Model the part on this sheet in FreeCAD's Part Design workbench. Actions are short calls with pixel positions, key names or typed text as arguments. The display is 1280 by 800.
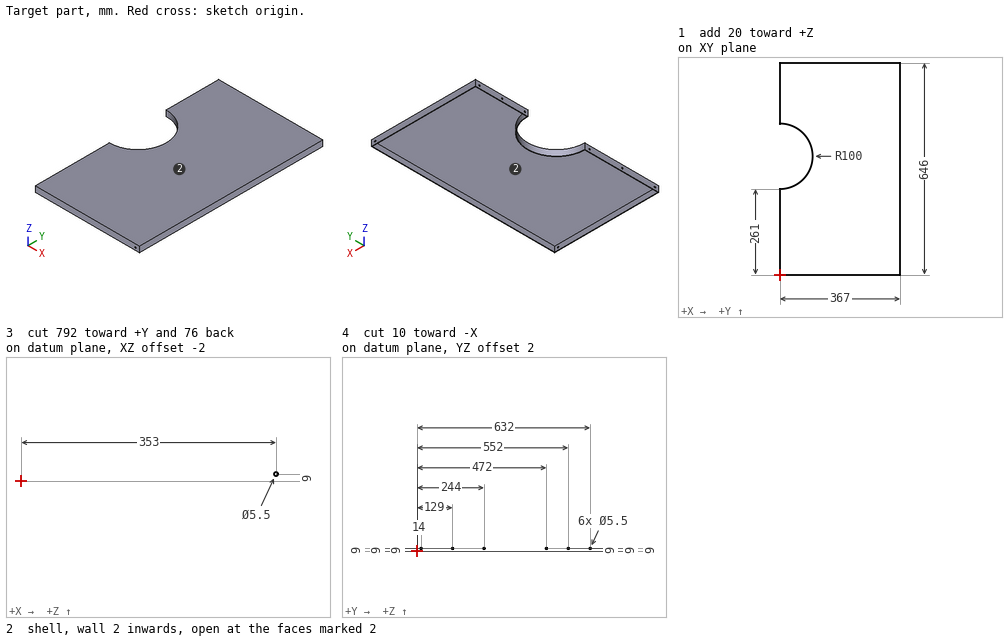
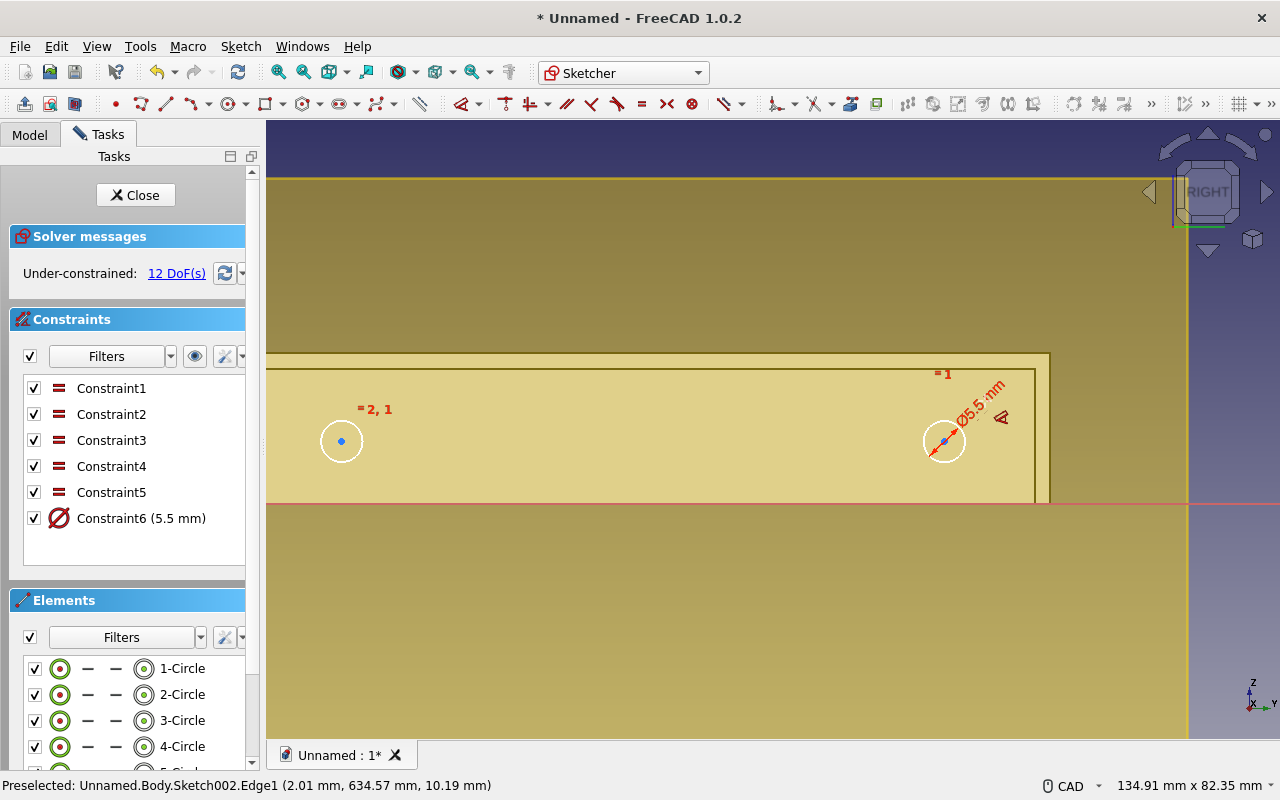
click(944, 442)
click(978, 473)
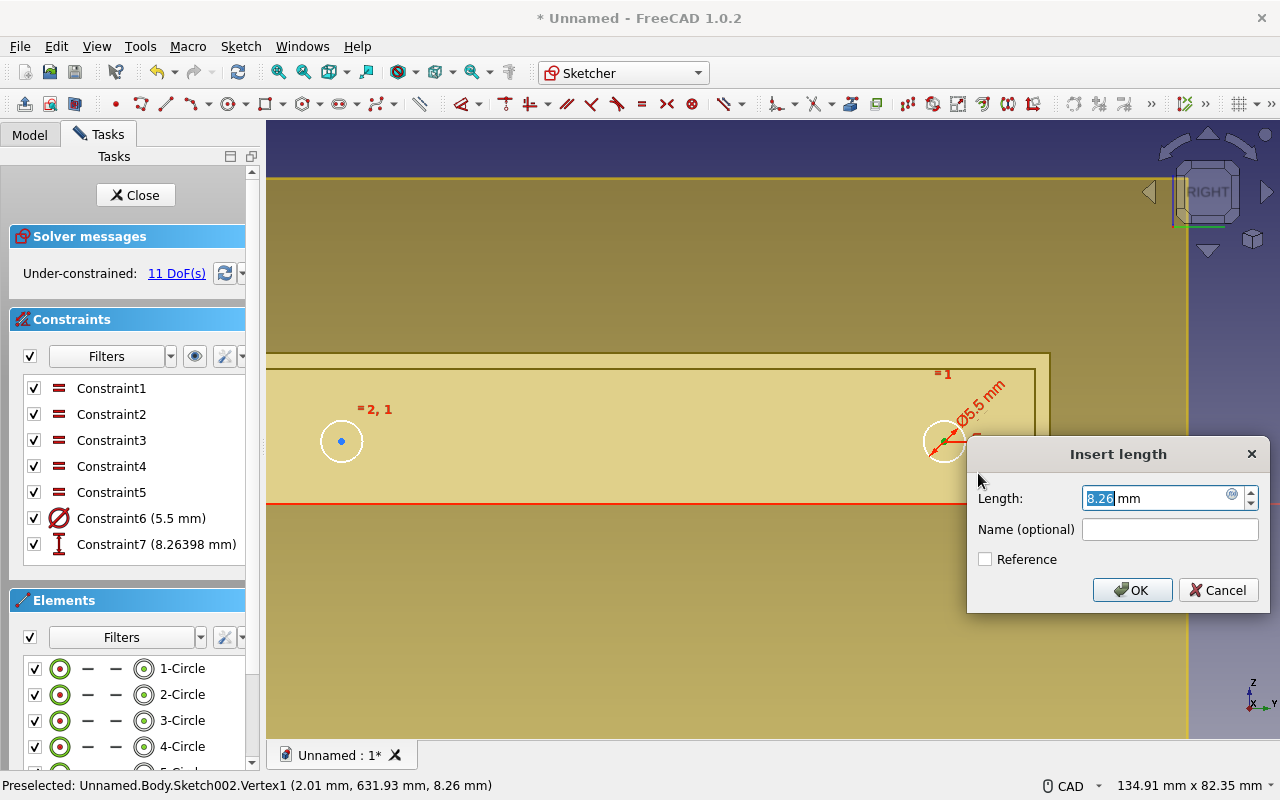
text(9)
key(Return)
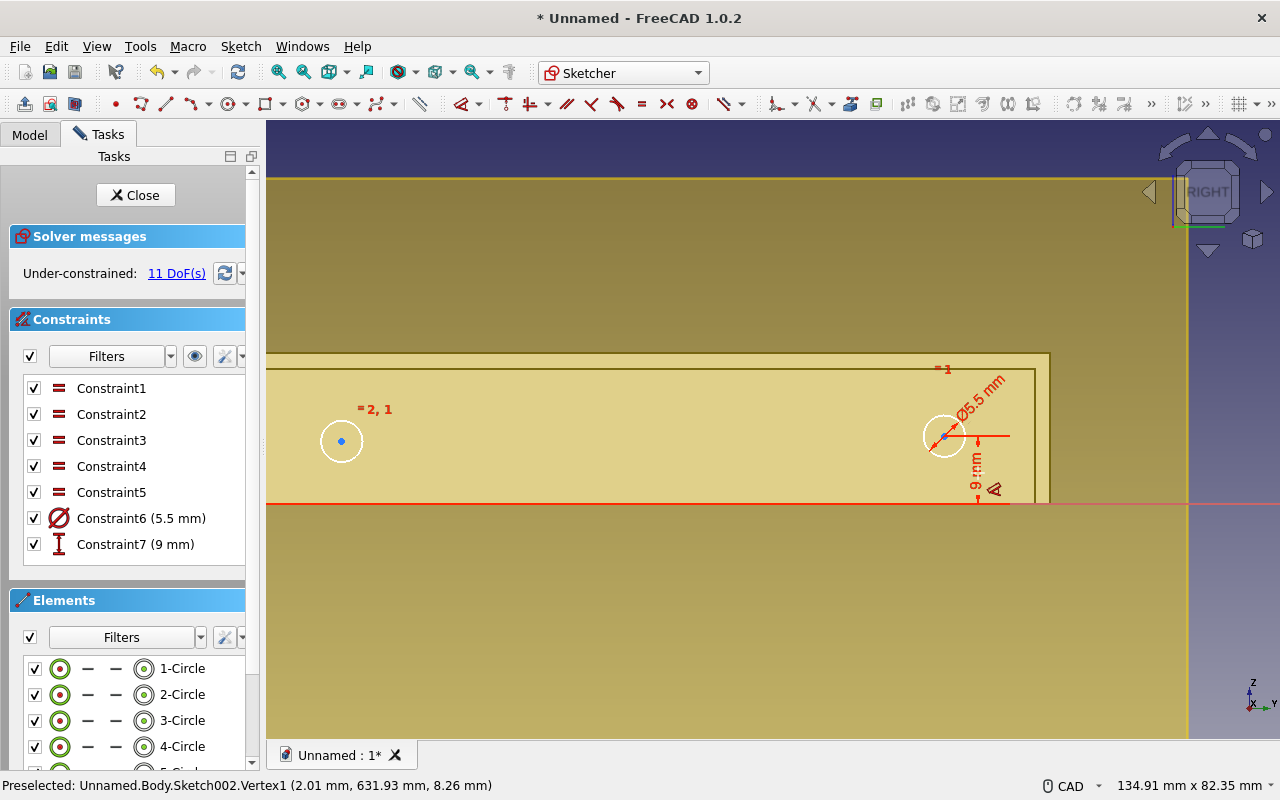
click(342, 441)
click(376, 473)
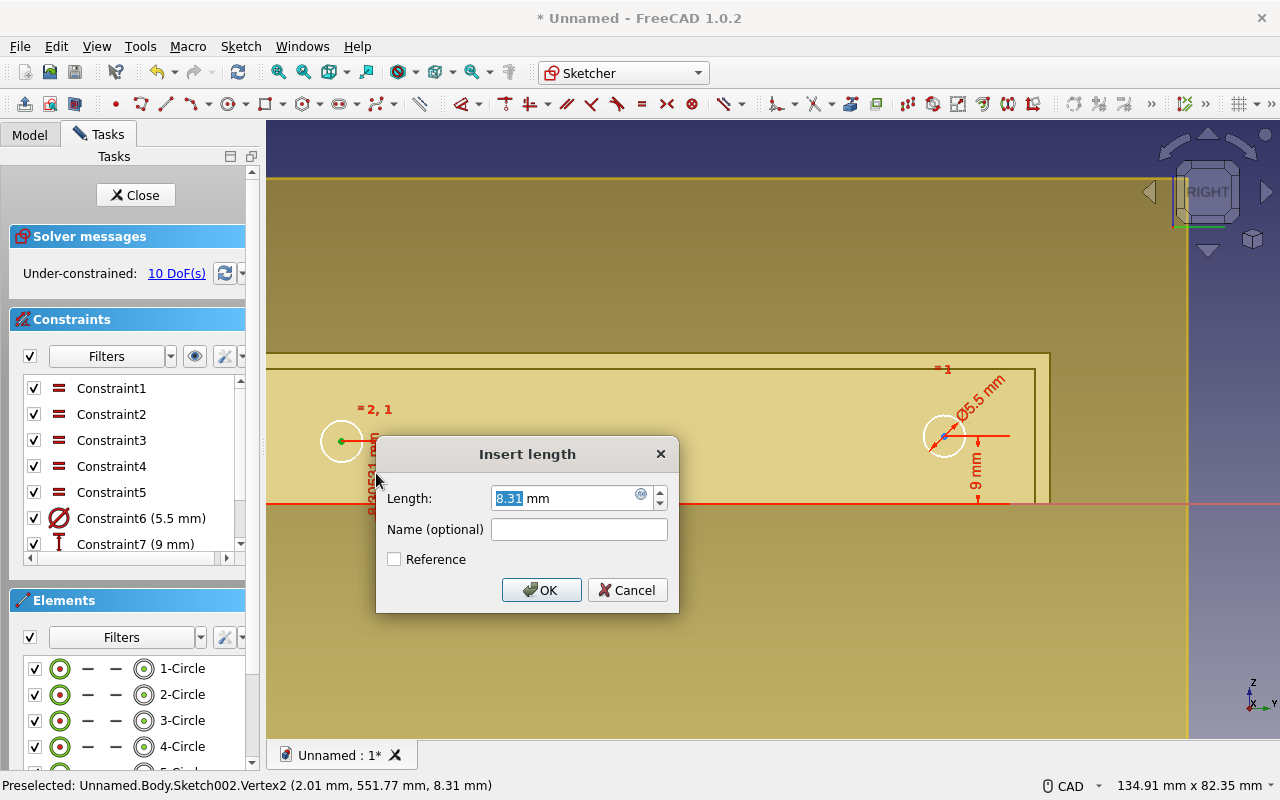
text(9)
key(Return)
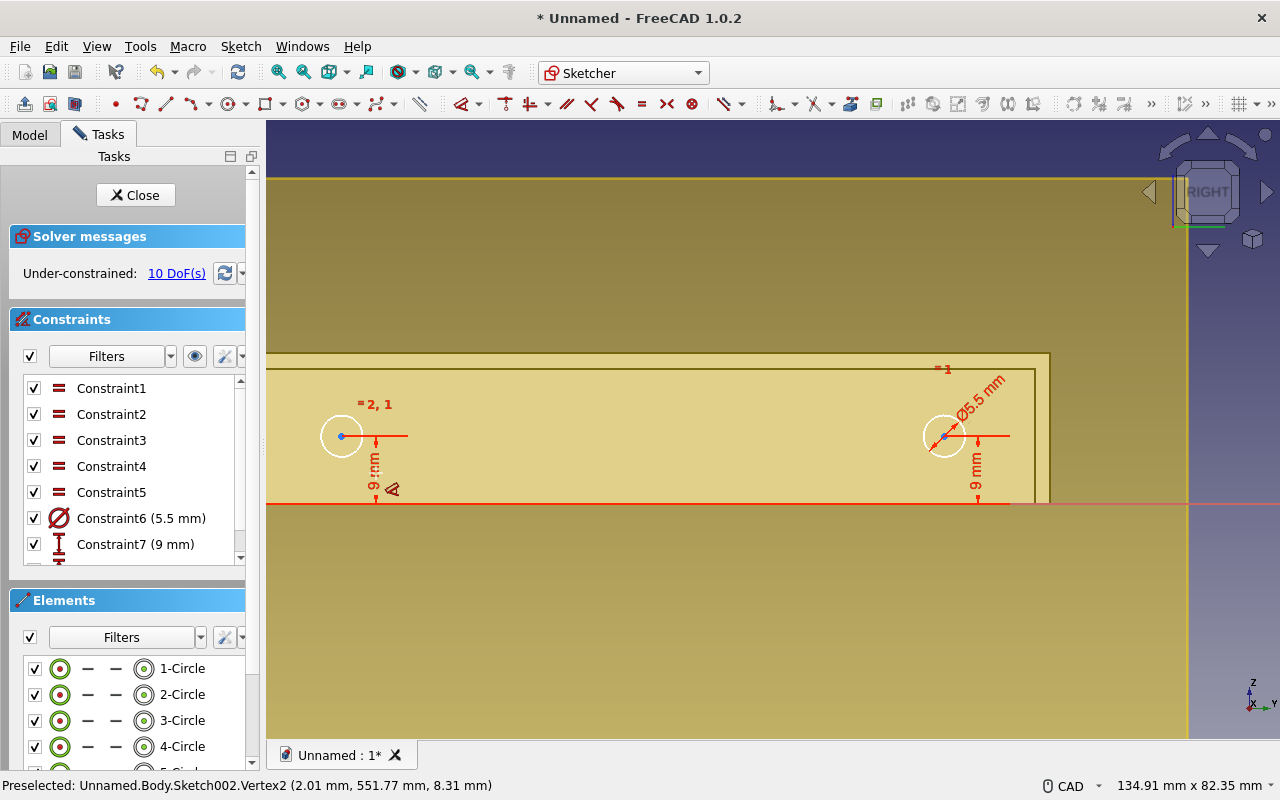
scroll(969, 426, down, 11)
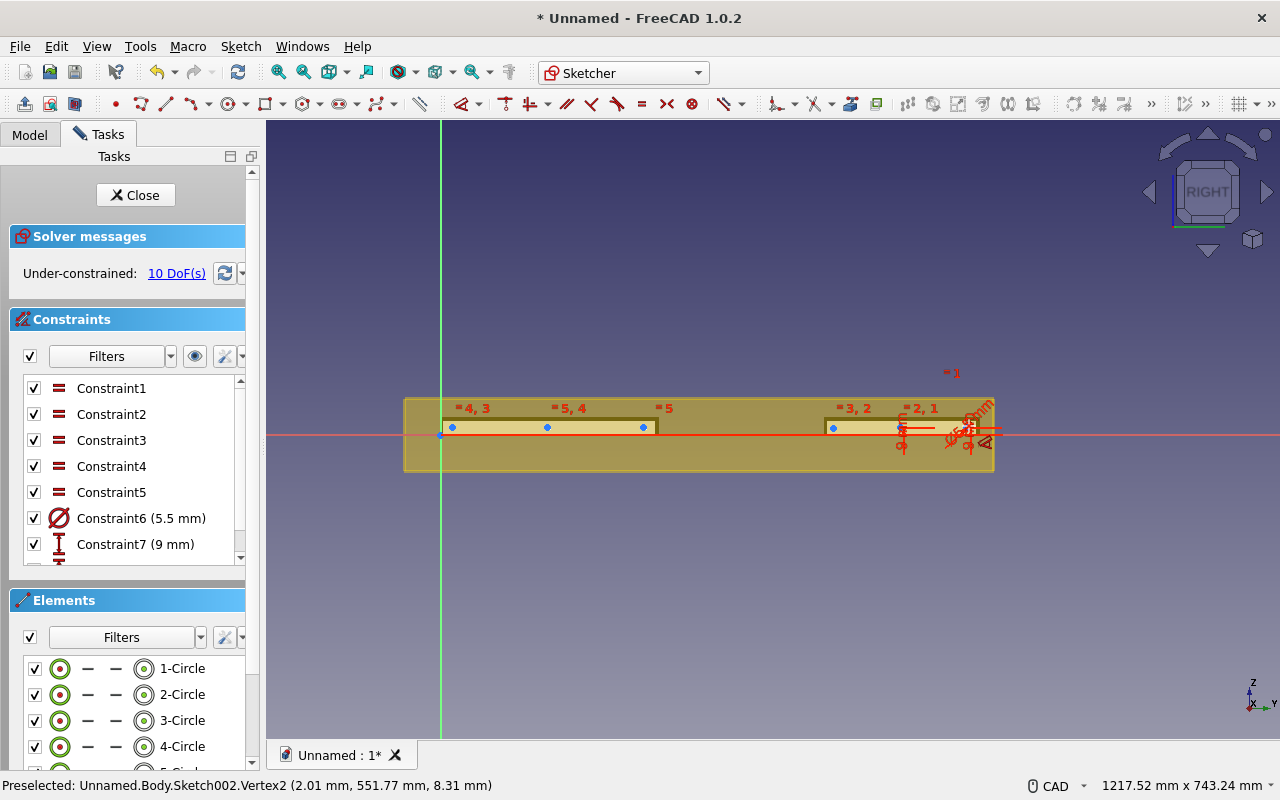
scroll(834, 428, up, 9)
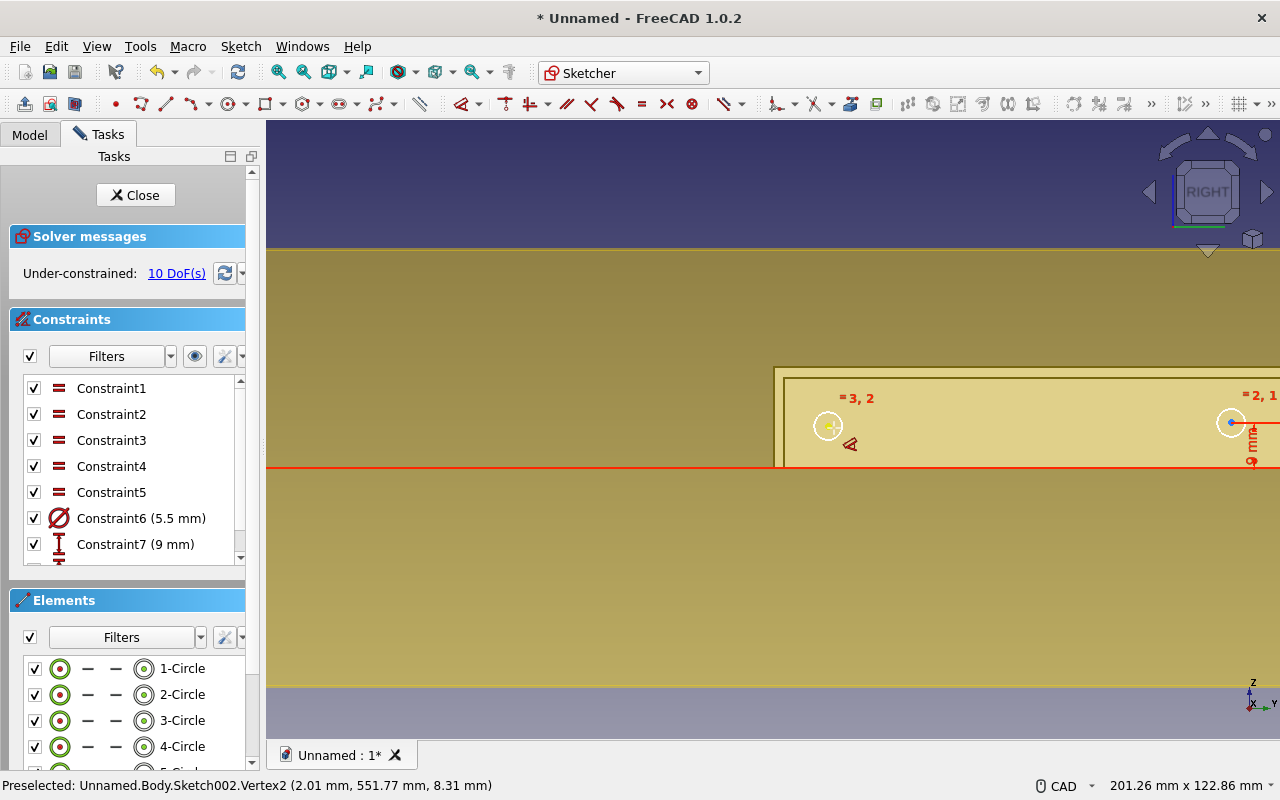
click(828, 426)
click(862, 447)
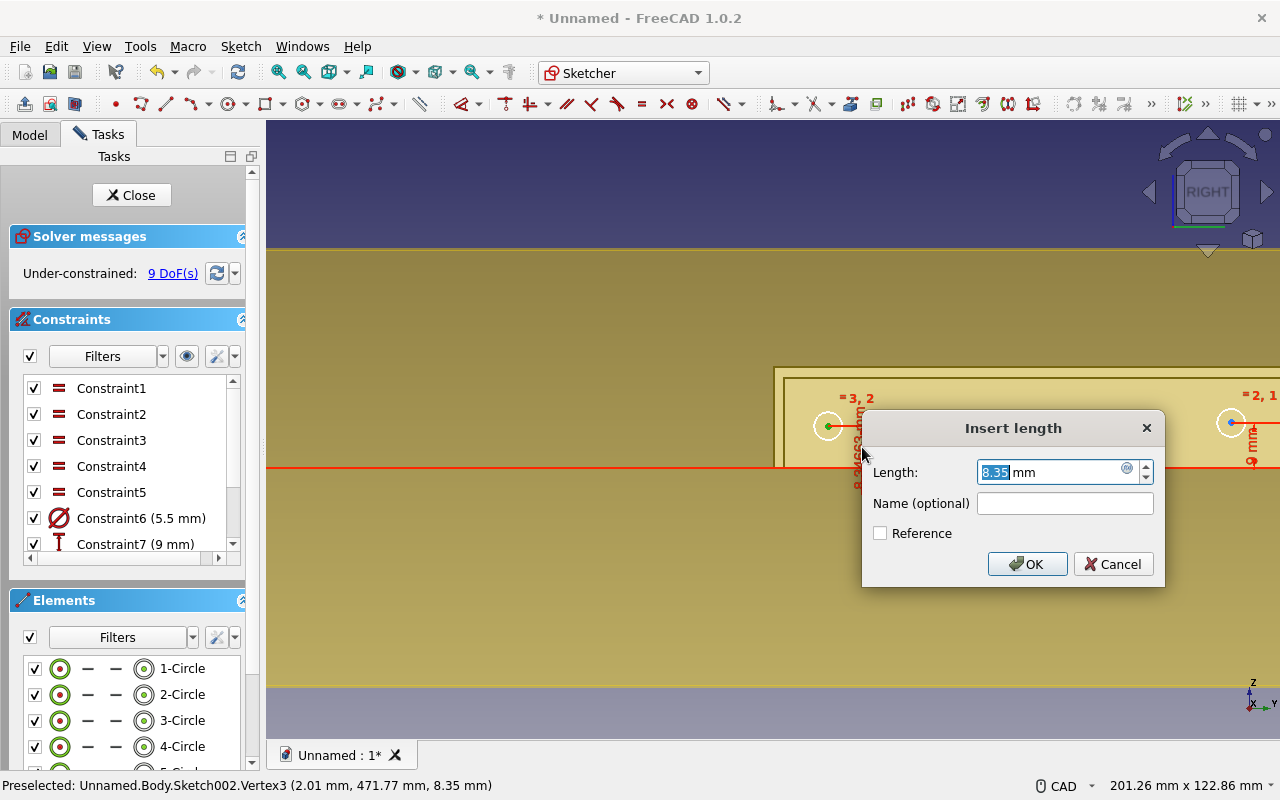
text(9)
key(Return)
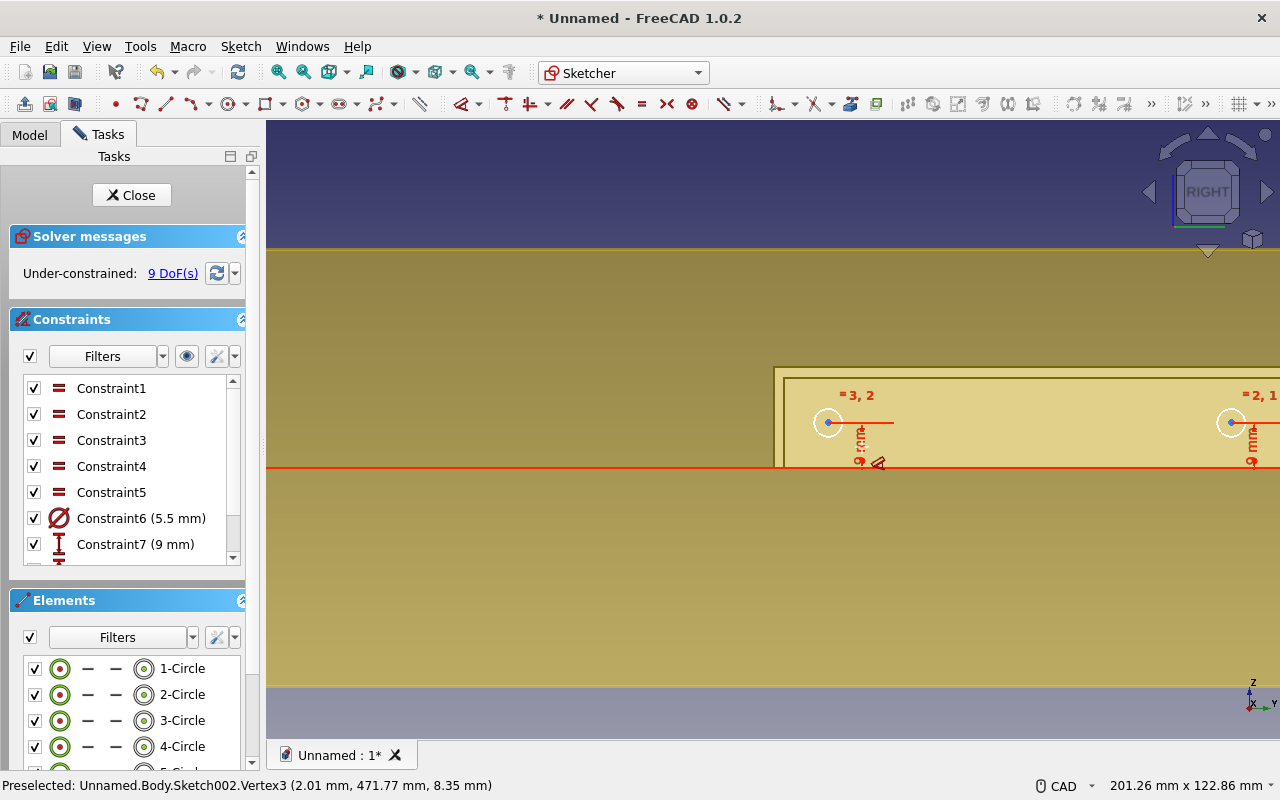
scroll(834, 428, down, 9)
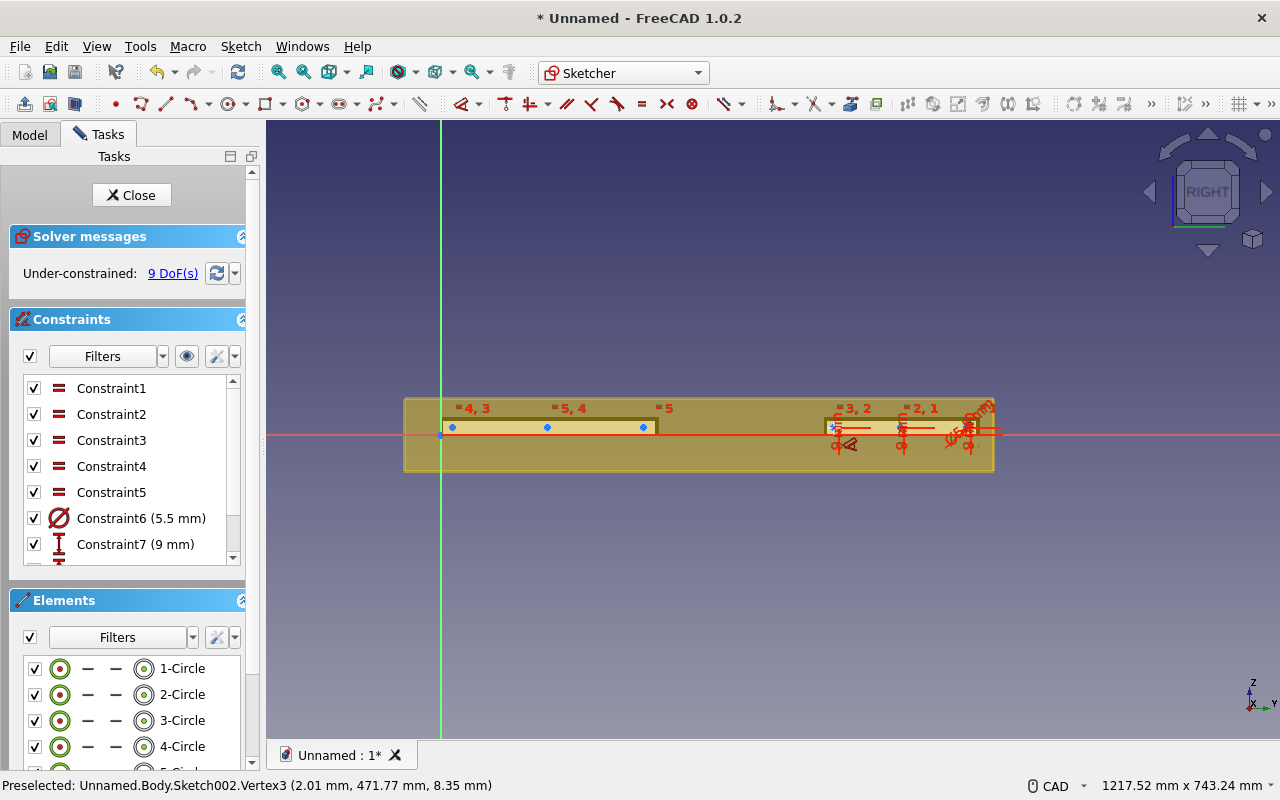
scroll(452, 428, up, 9)